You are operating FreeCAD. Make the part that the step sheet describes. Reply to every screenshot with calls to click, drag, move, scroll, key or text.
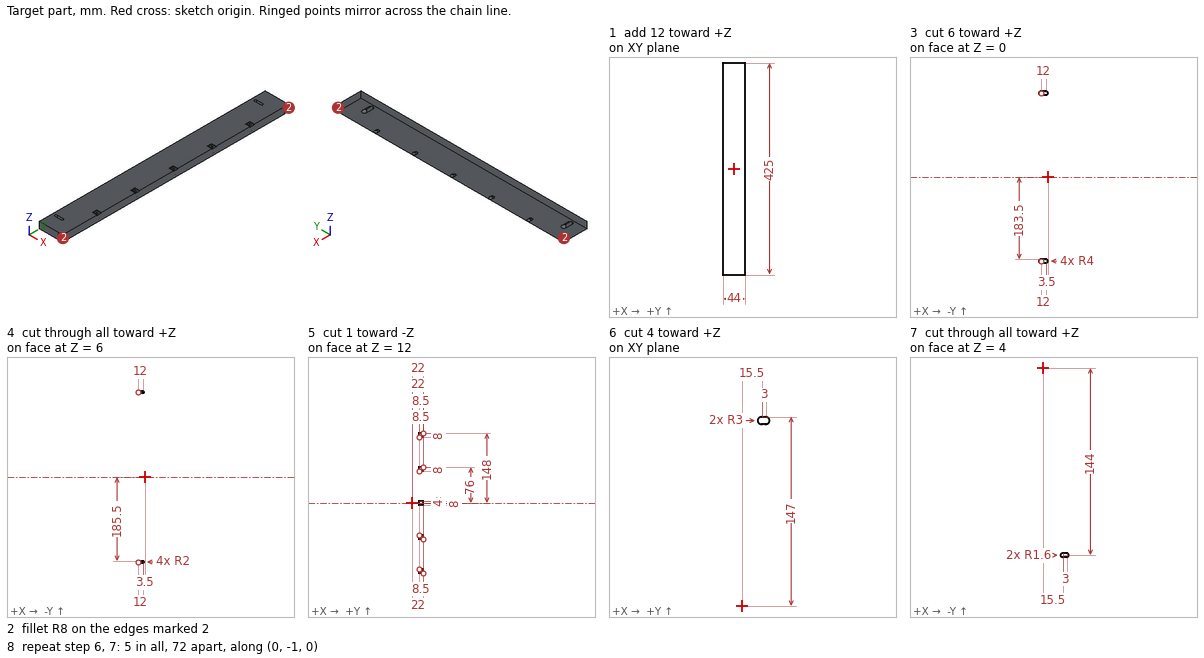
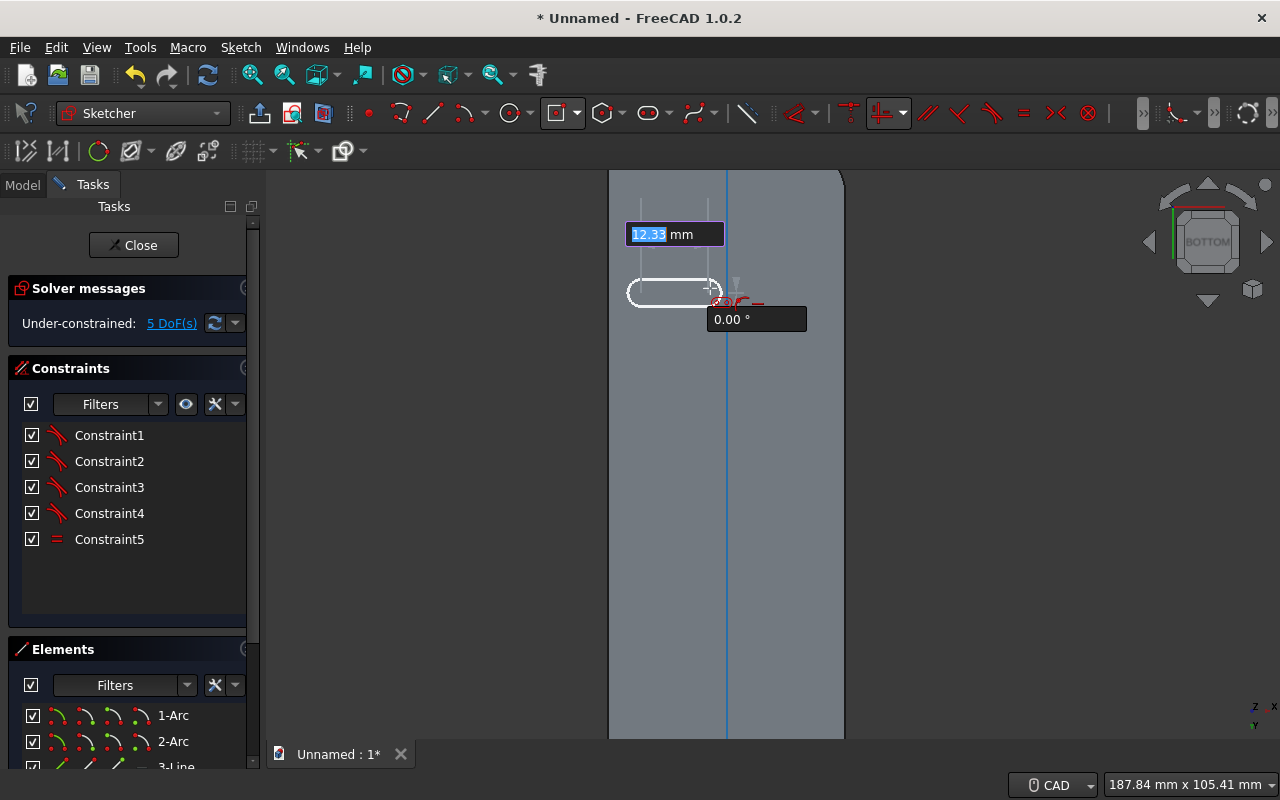
click(708, 287)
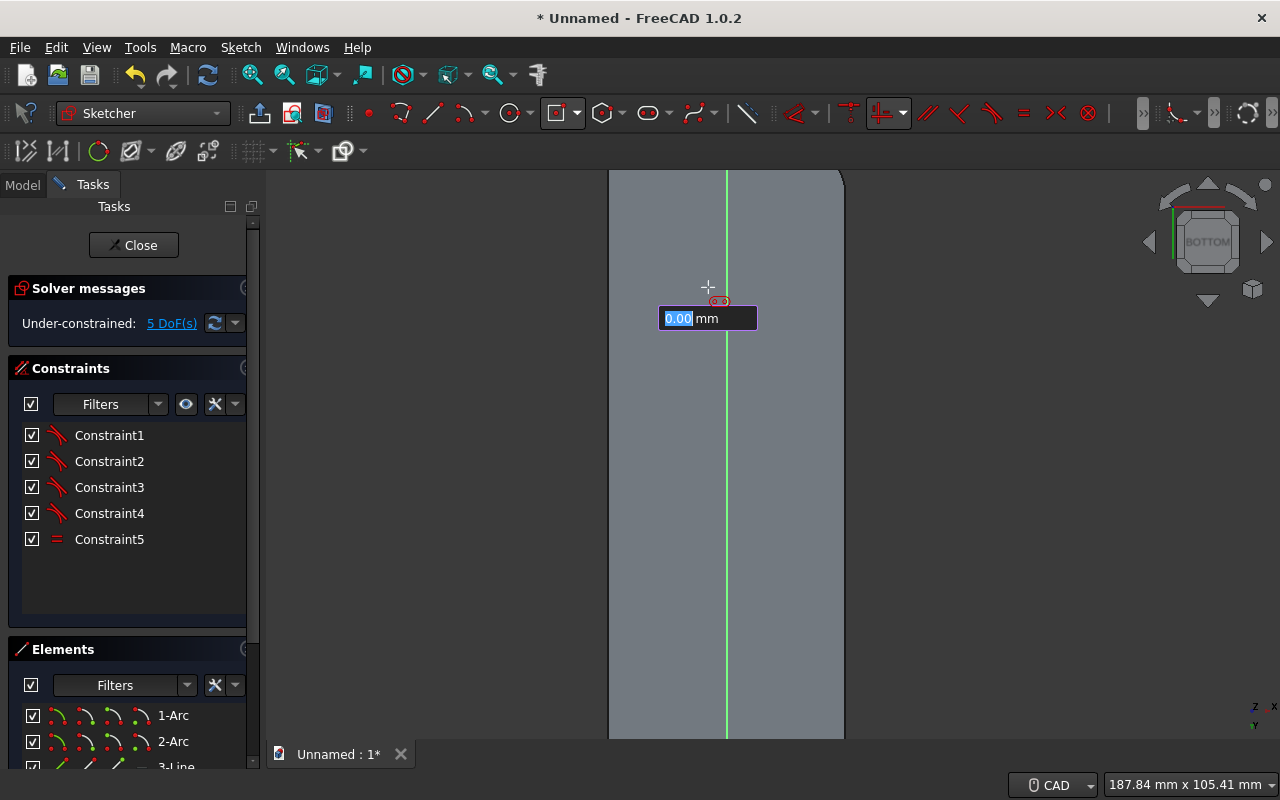
click(675, 262)
key(Escape)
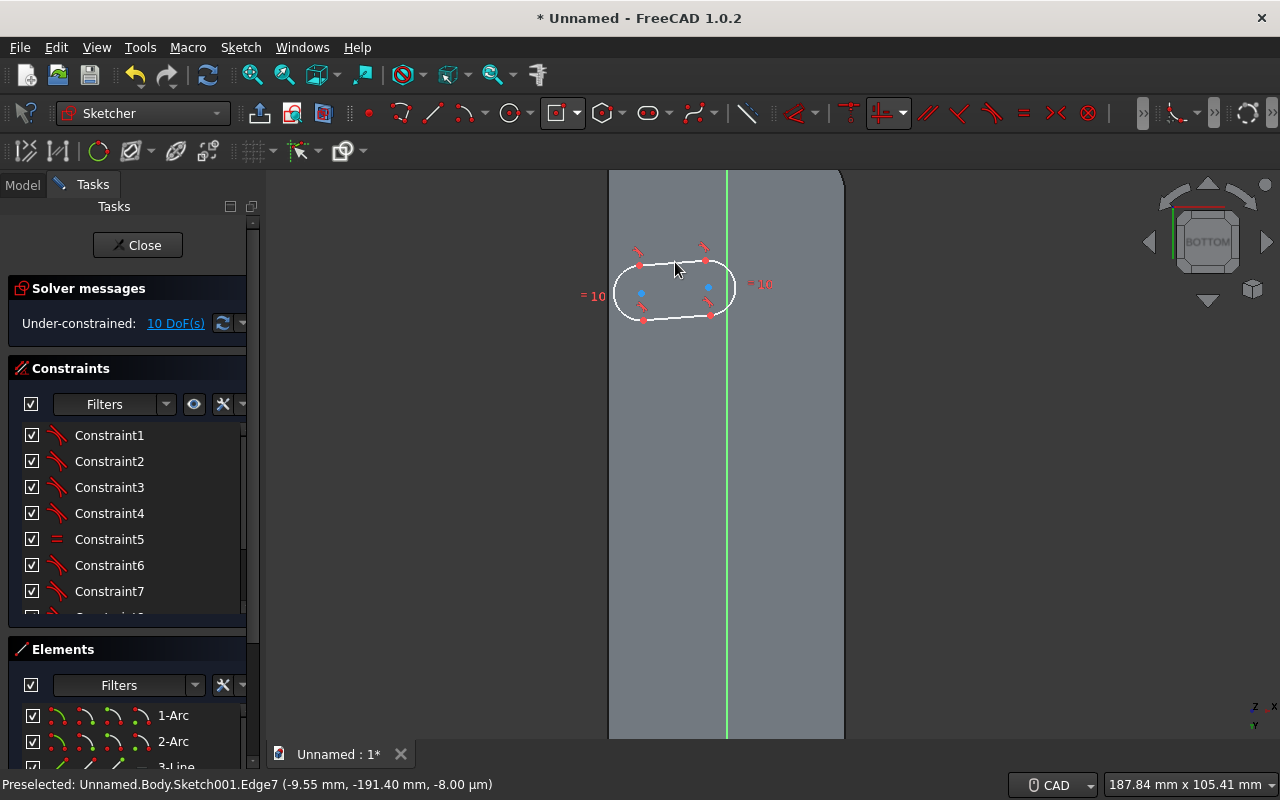
scroll(710, 288, down, 9)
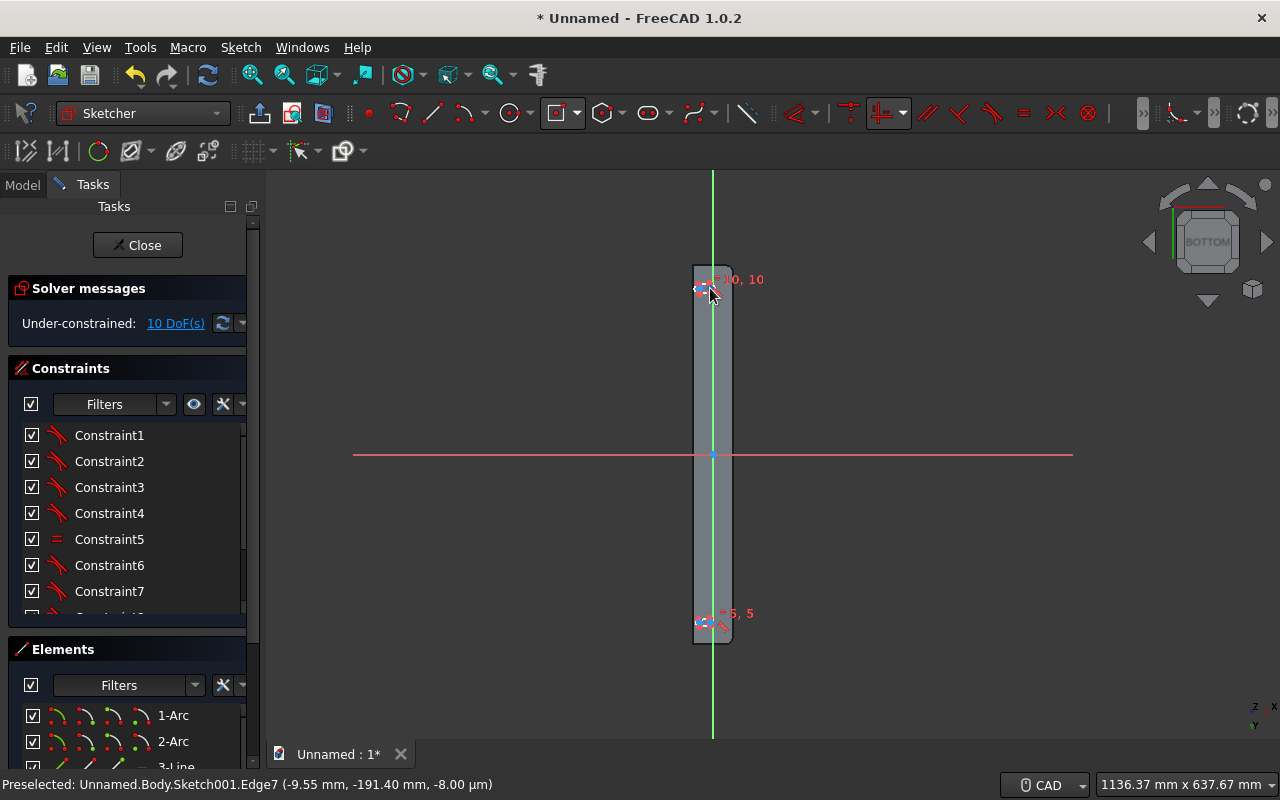
scroll(702, 620, up, 8)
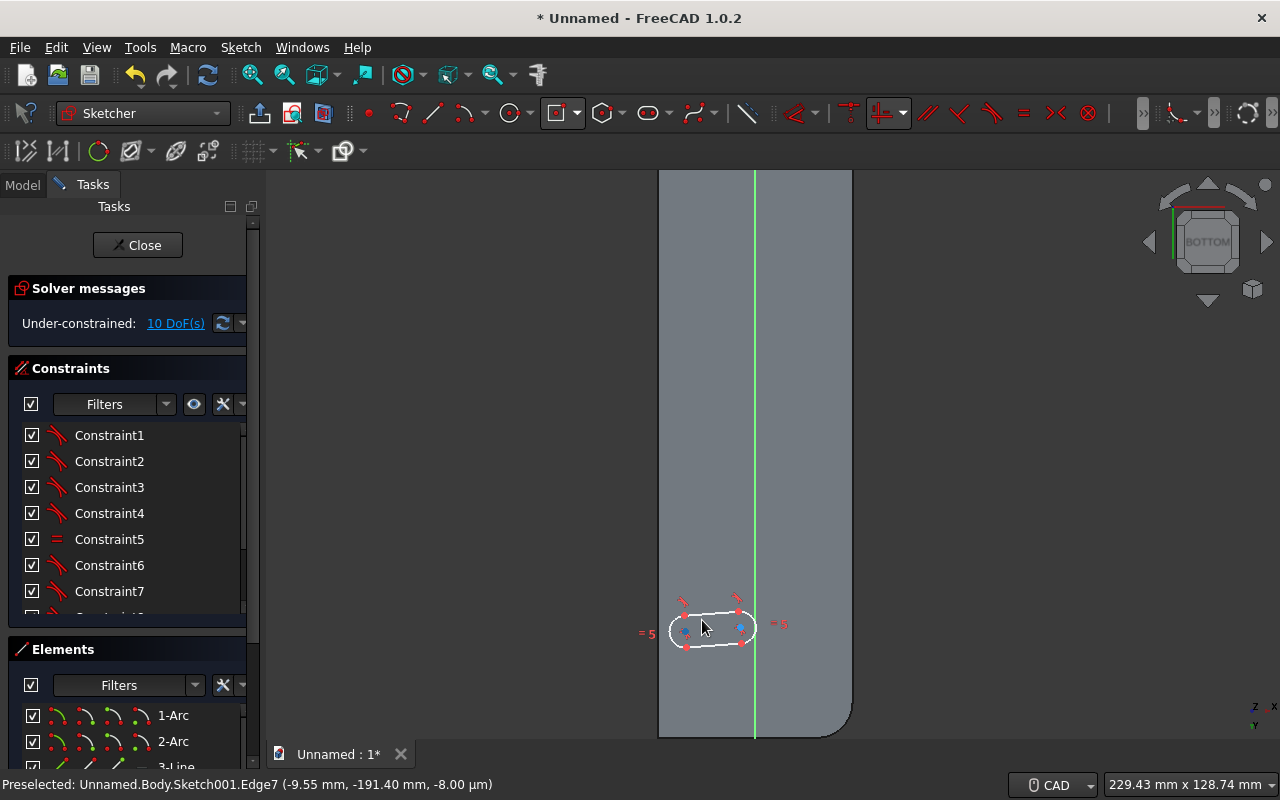
click(701, 615)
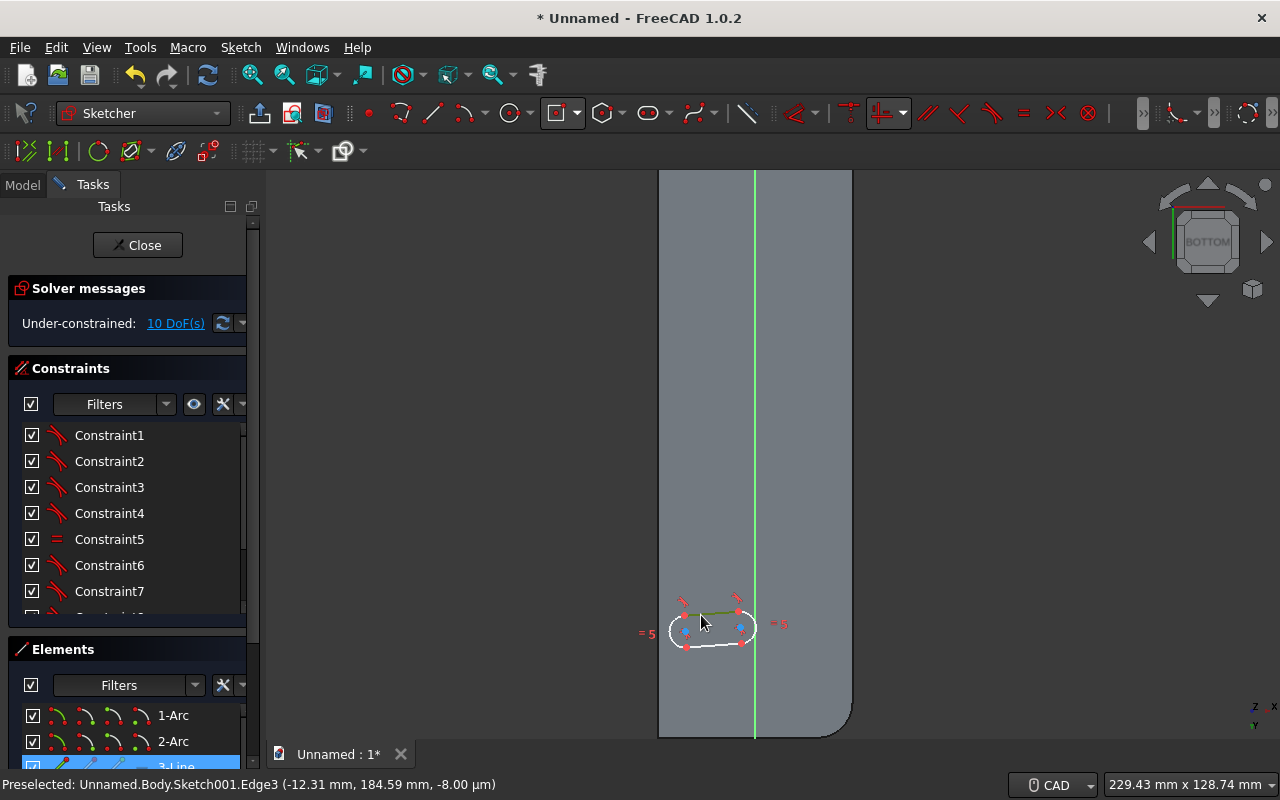
click(906, 114)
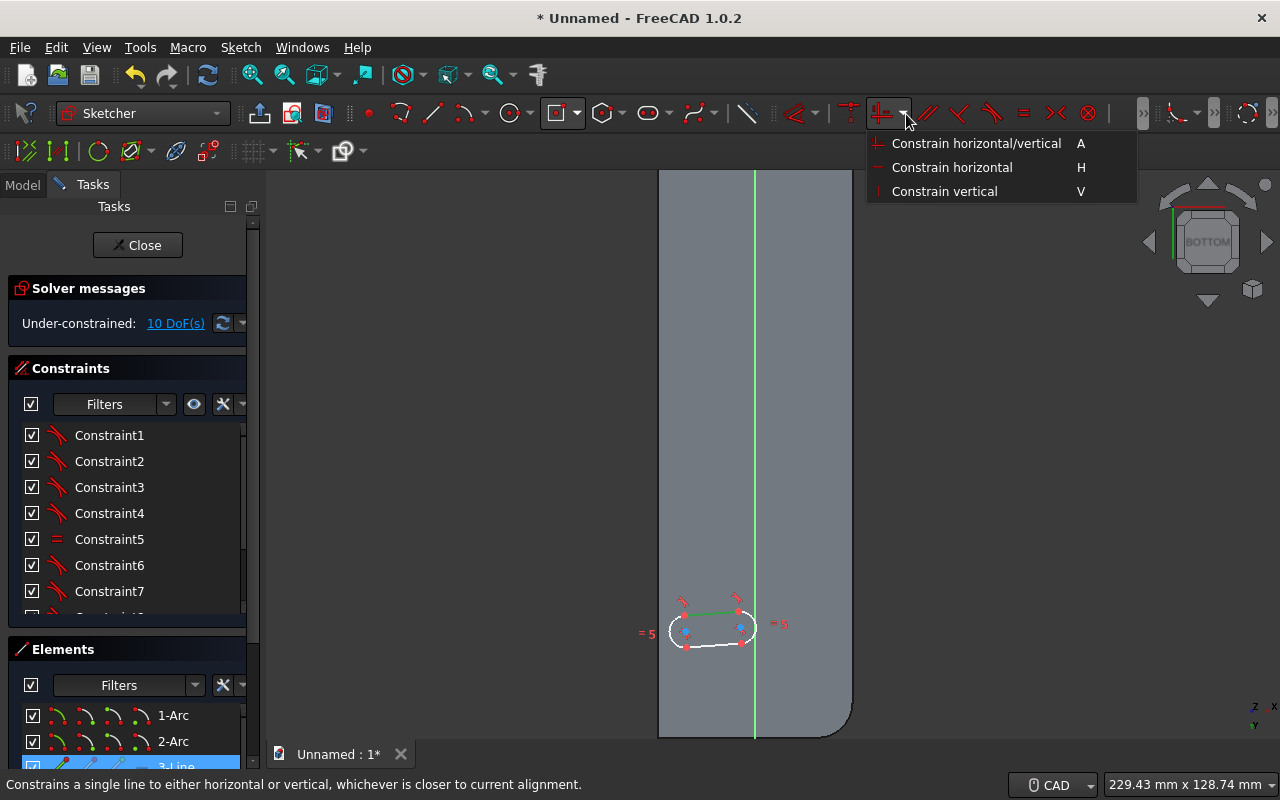
click(1002, 167)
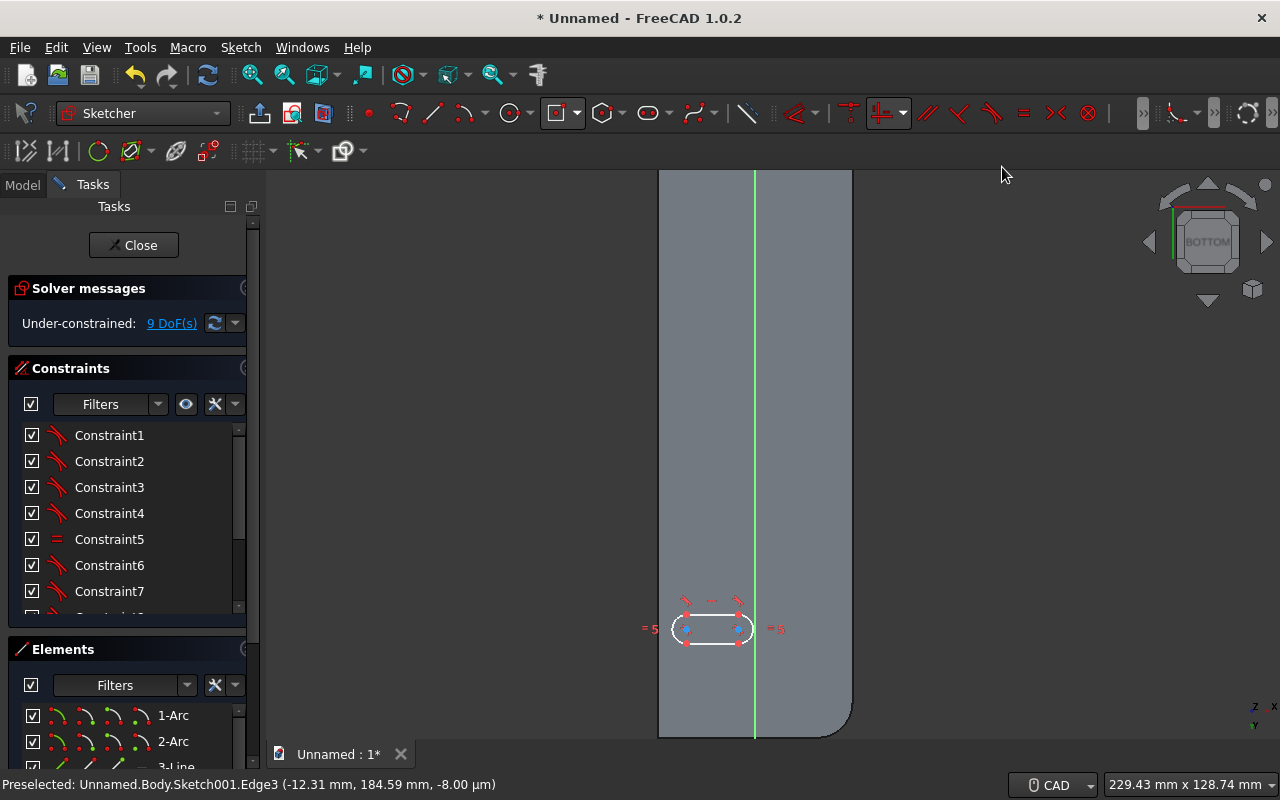
scroll(702, 620, down, 8)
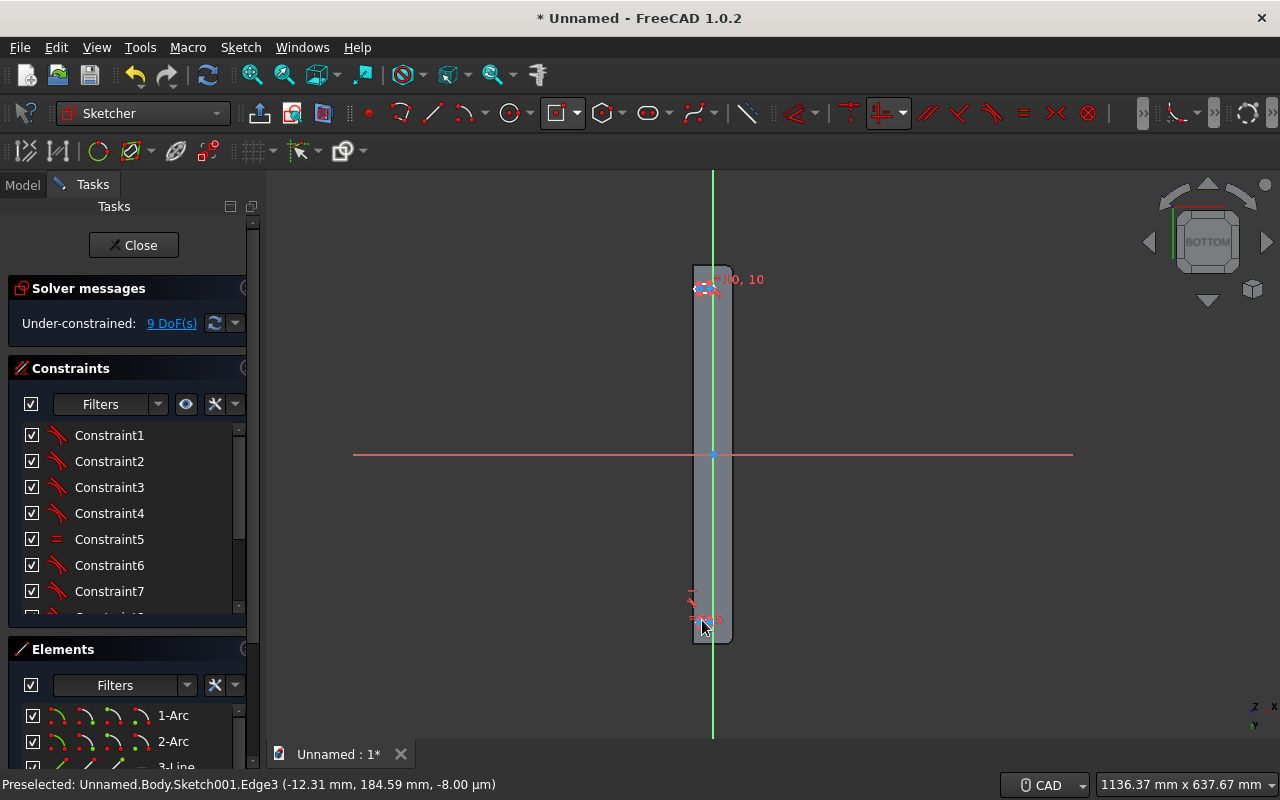
scroll(702, 284, up, 8)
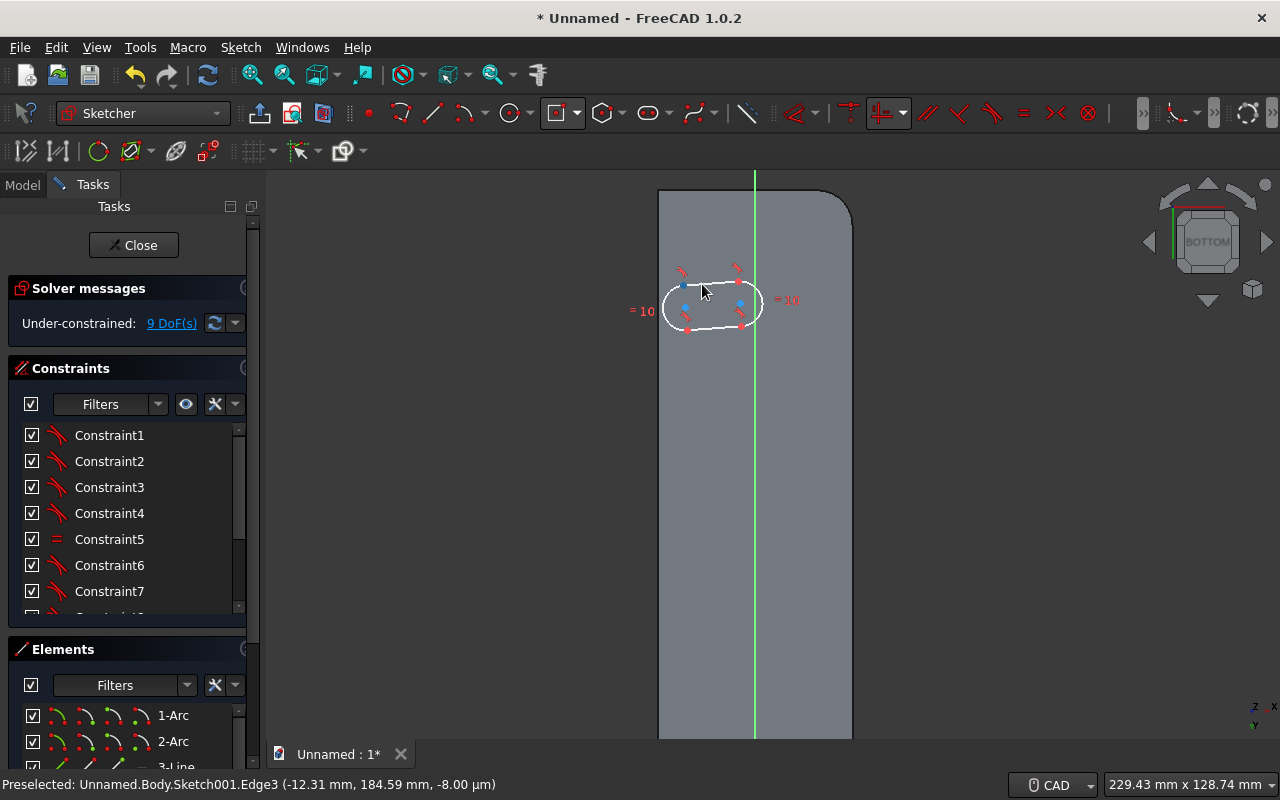
click(700, 284)